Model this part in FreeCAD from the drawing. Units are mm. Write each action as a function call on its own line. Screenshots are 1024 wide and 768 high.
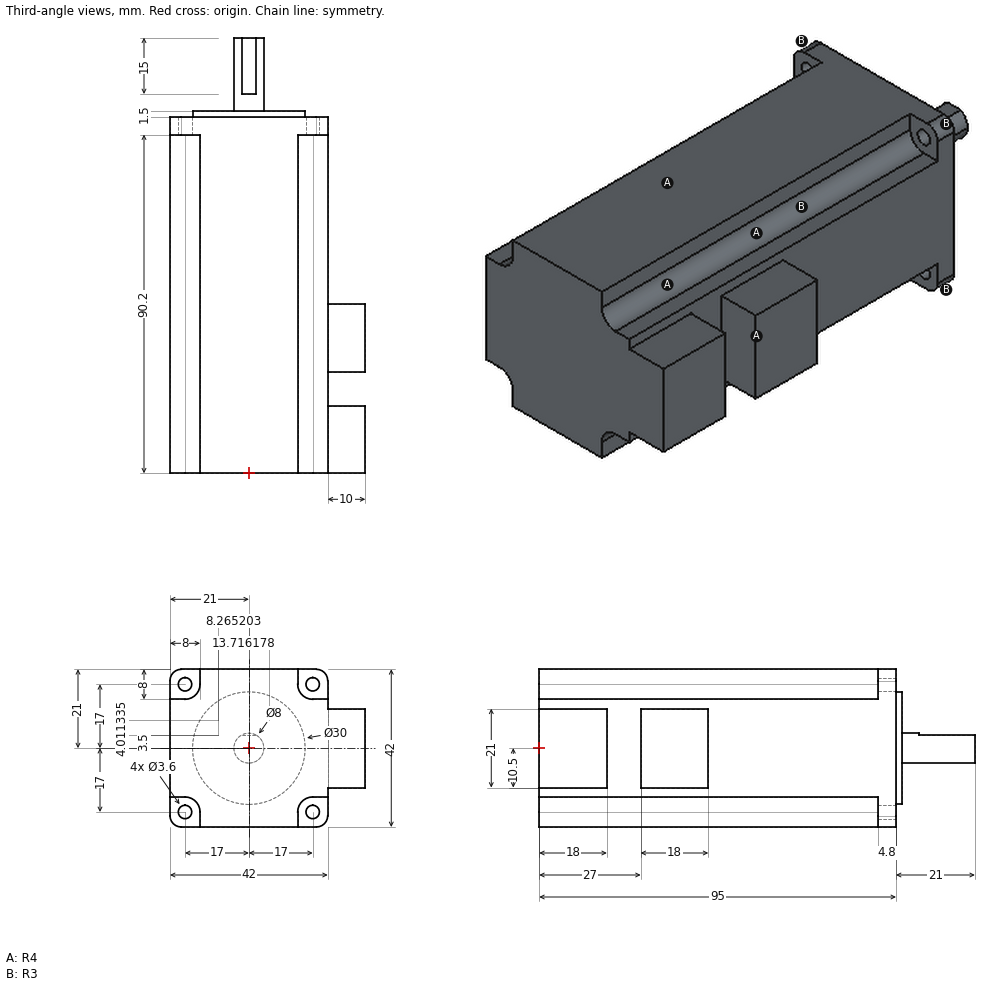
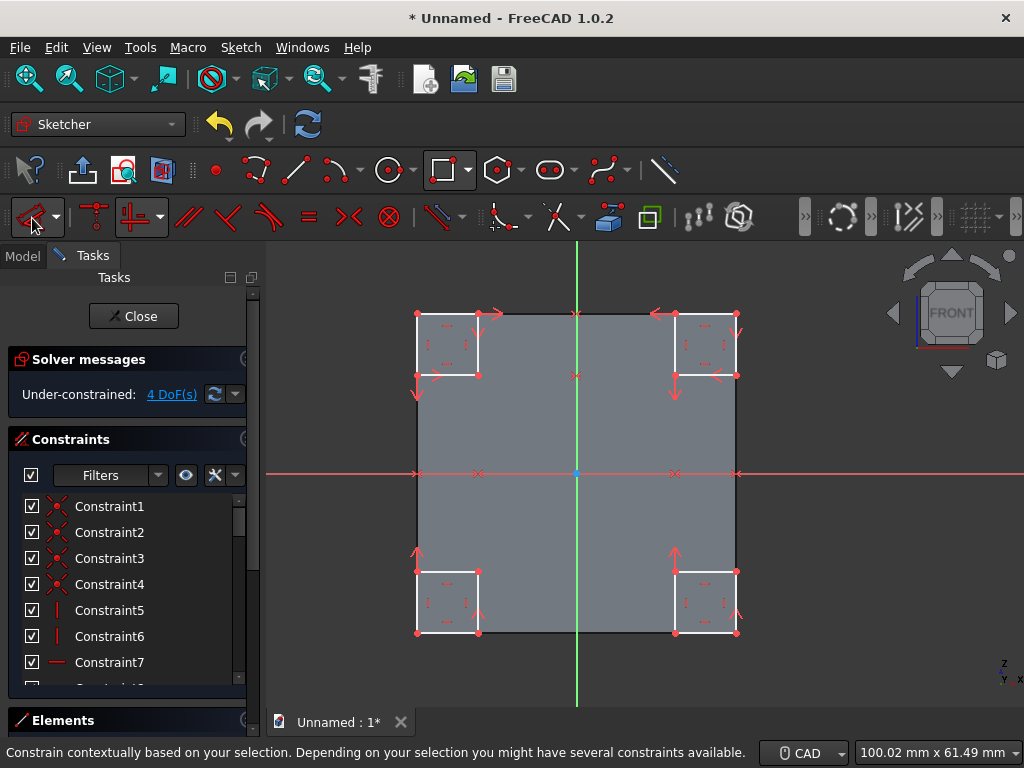
click(417, 332)
click(383, 345)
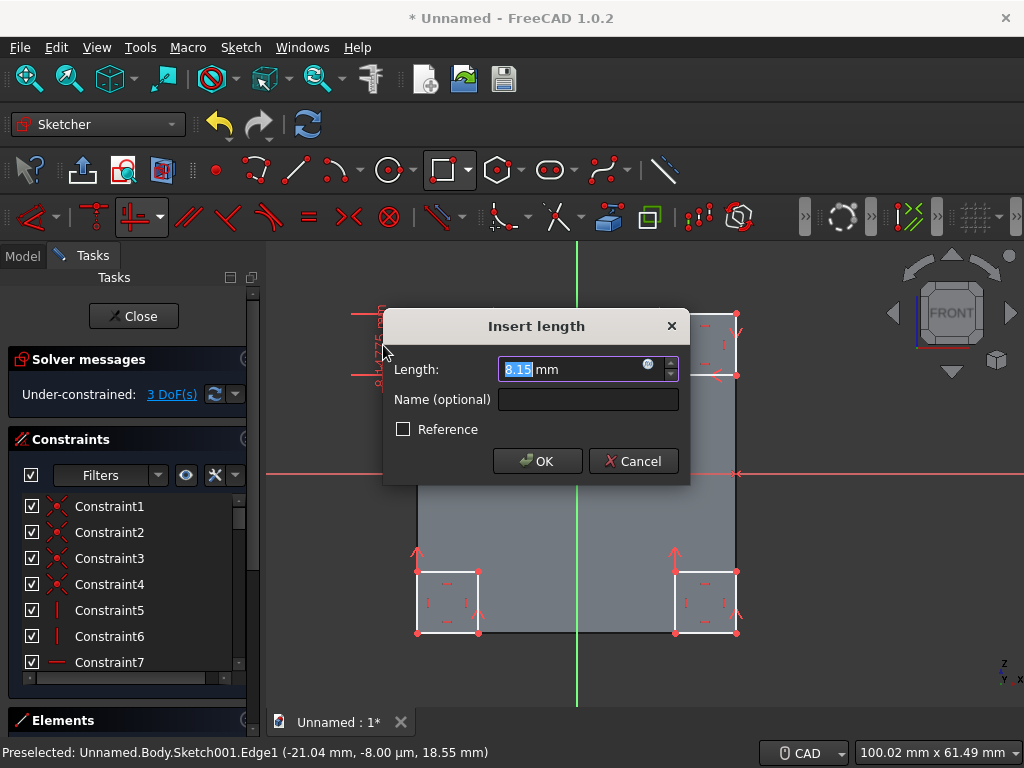
text(8)
key(Return)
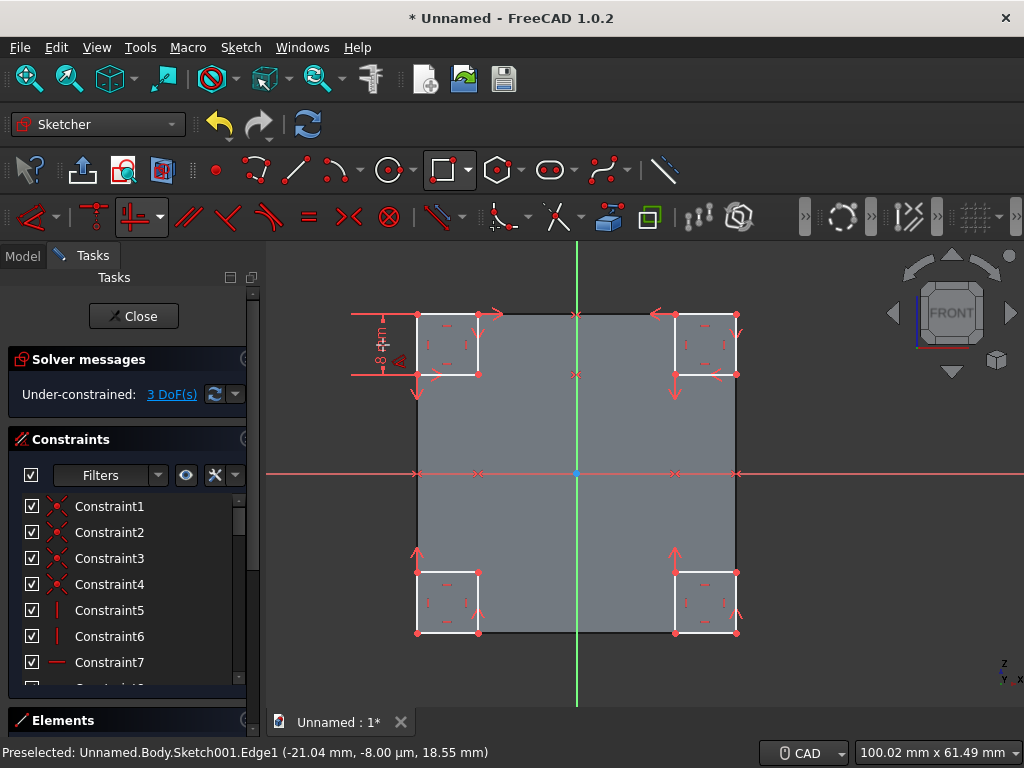
click(435, 375)
click(462, 341)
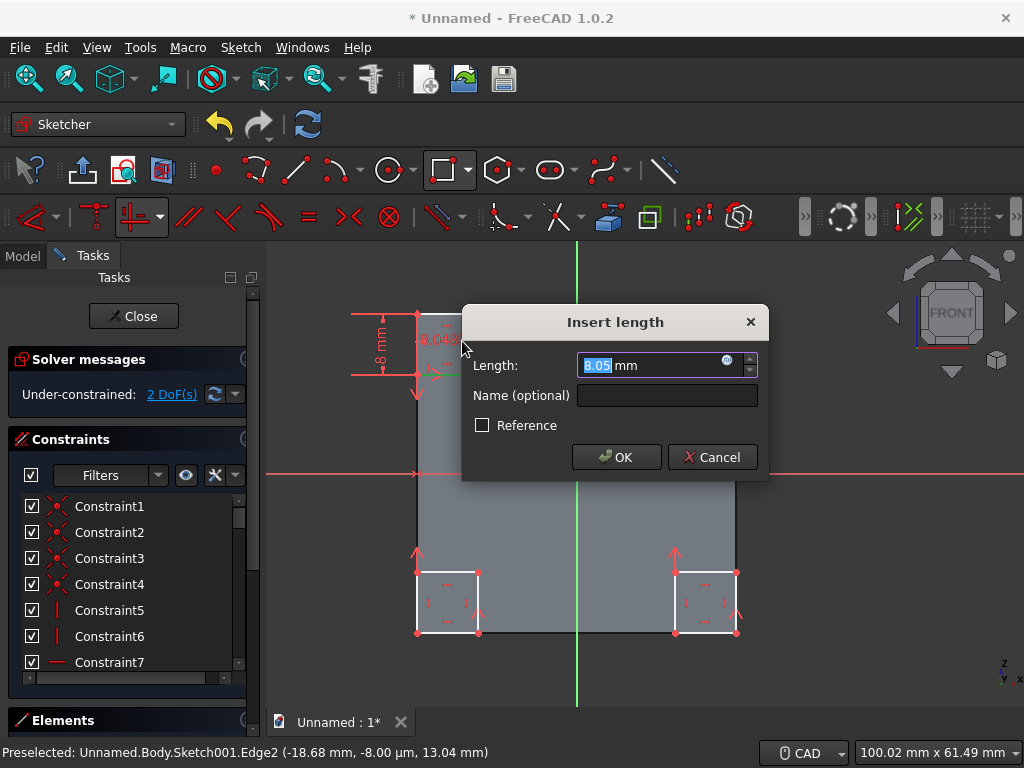
text(8)
key(Return)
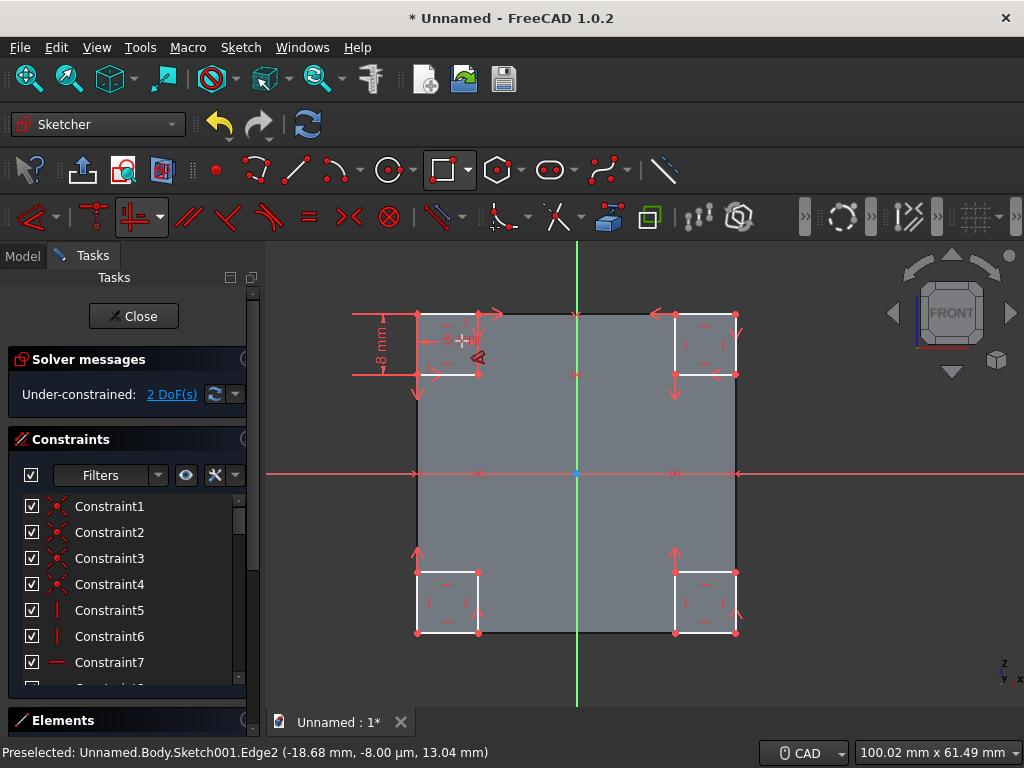
click(417, 314)
click(497, 280)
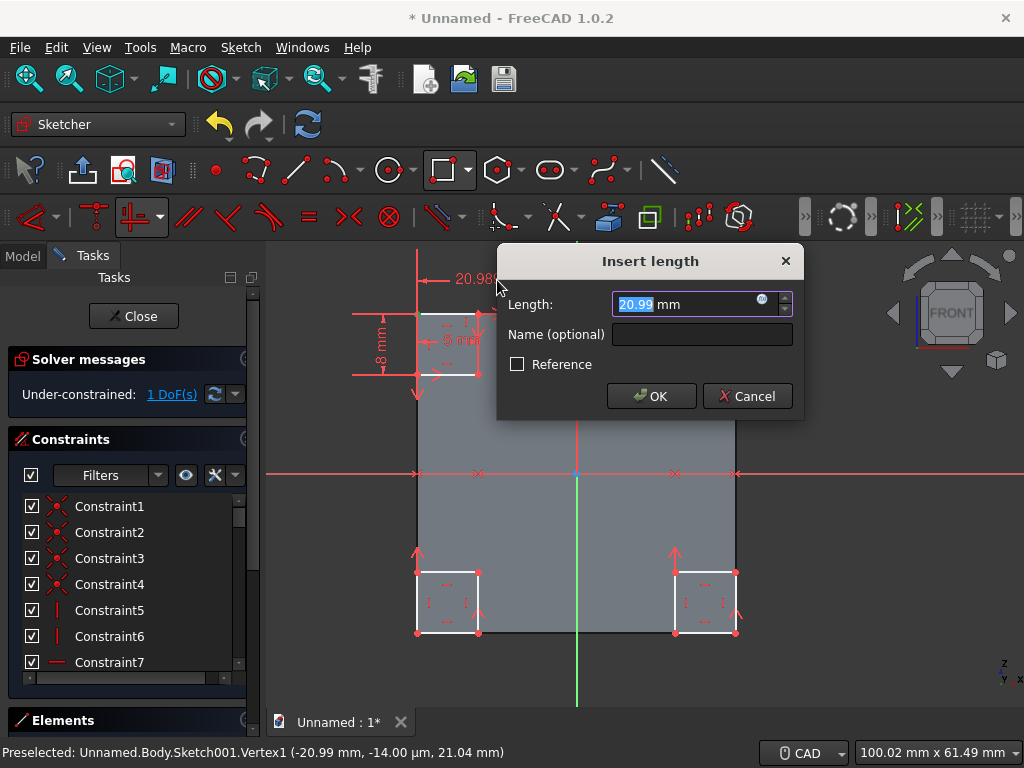
text(21)
key(Return)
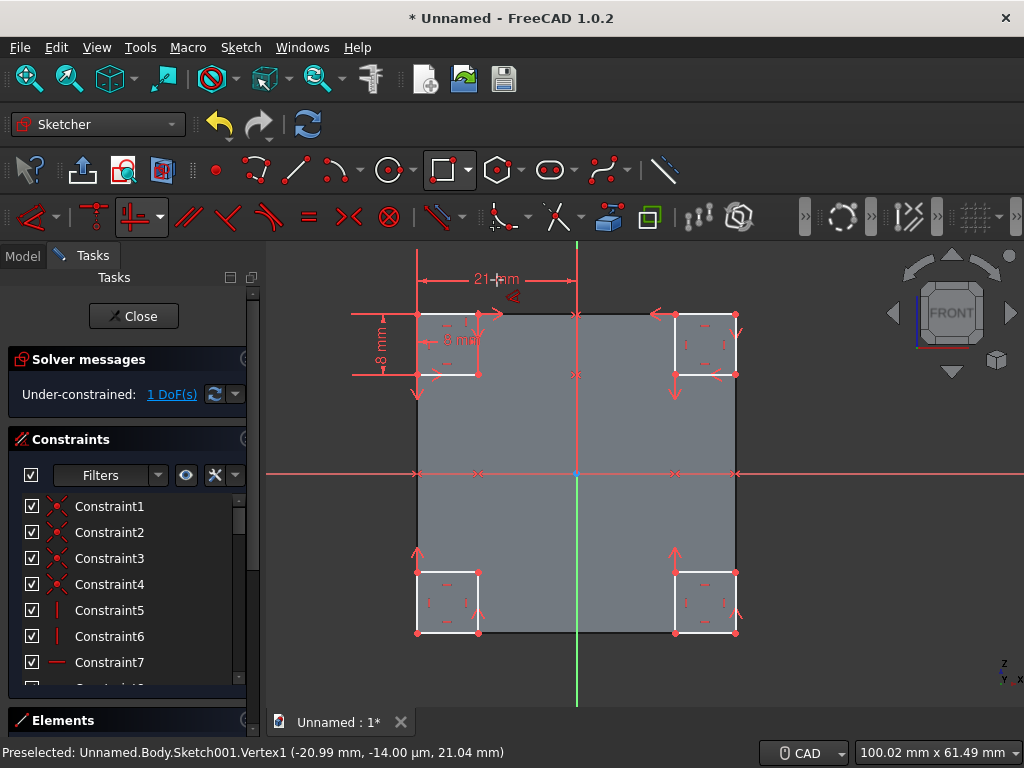
click(417, 314)
click(383, 394)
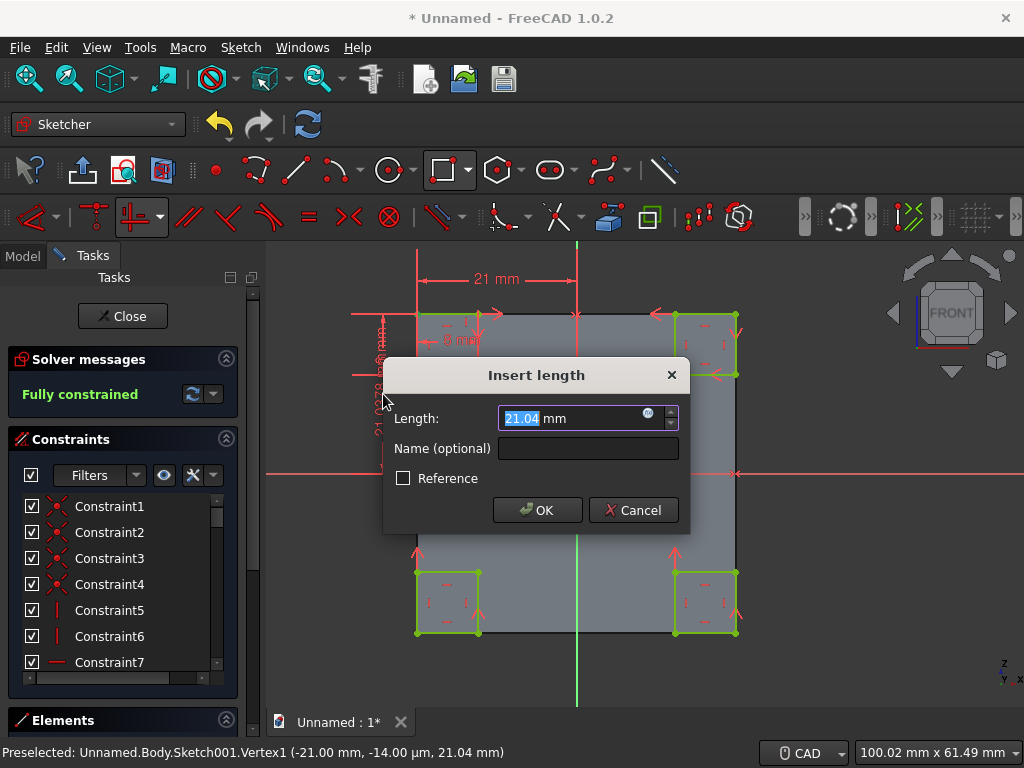
text(21)
key(Return)
key(Escape)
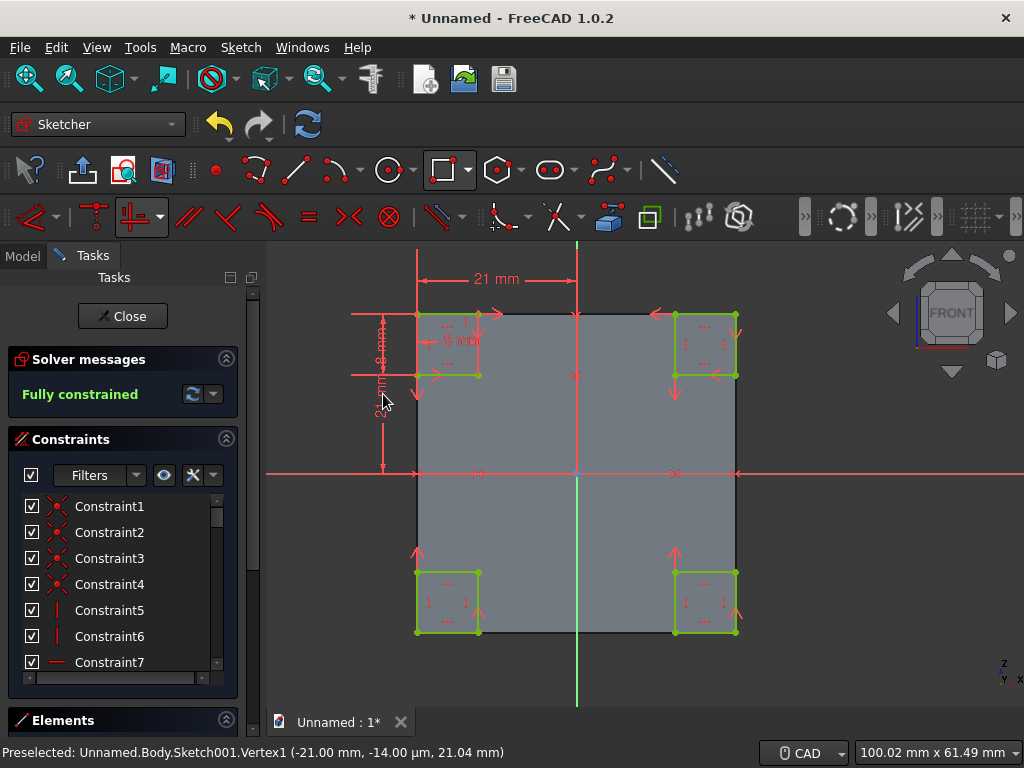
click(123, 316)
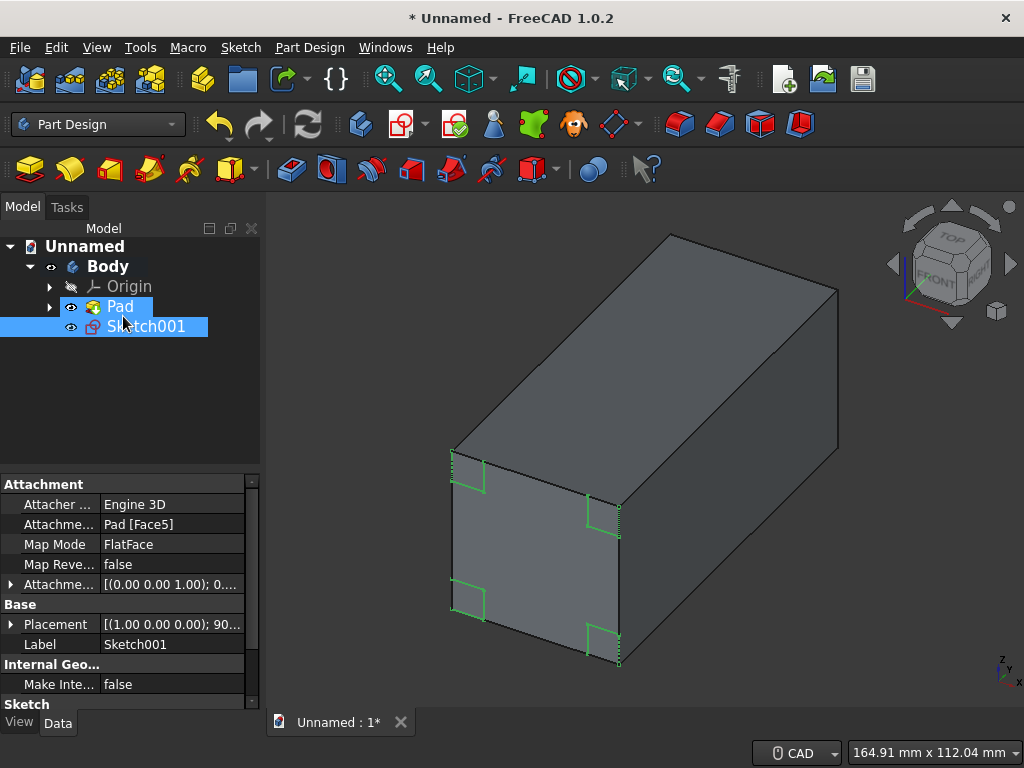
click(292, 170)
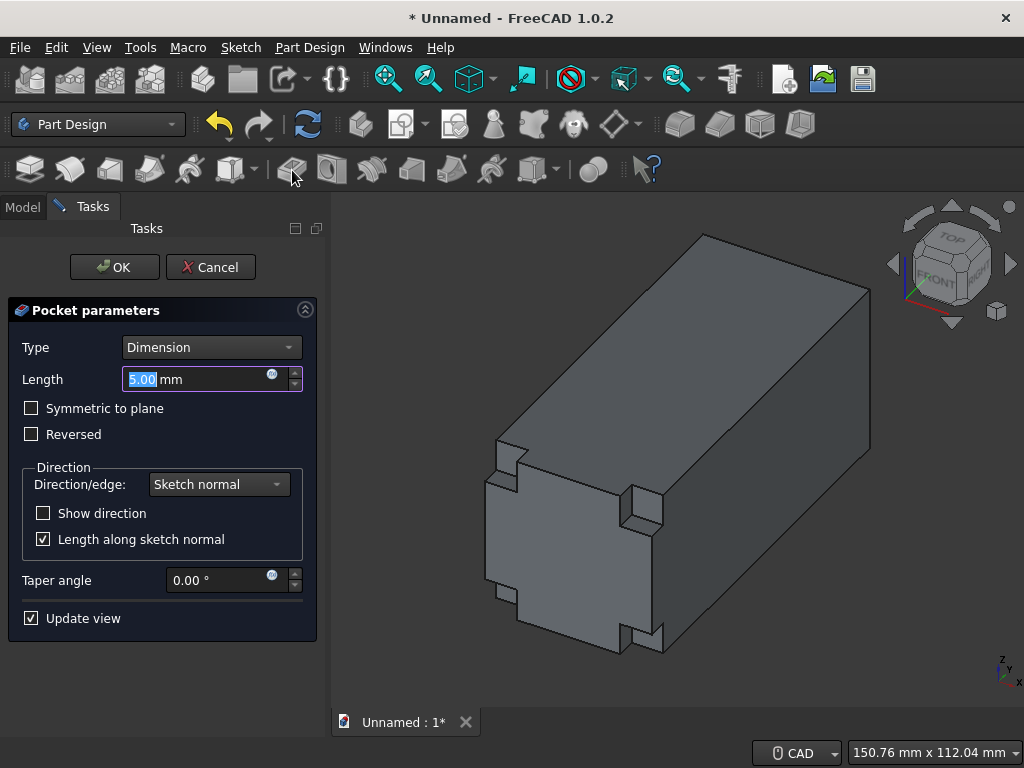
text(90.2)
key(Tab)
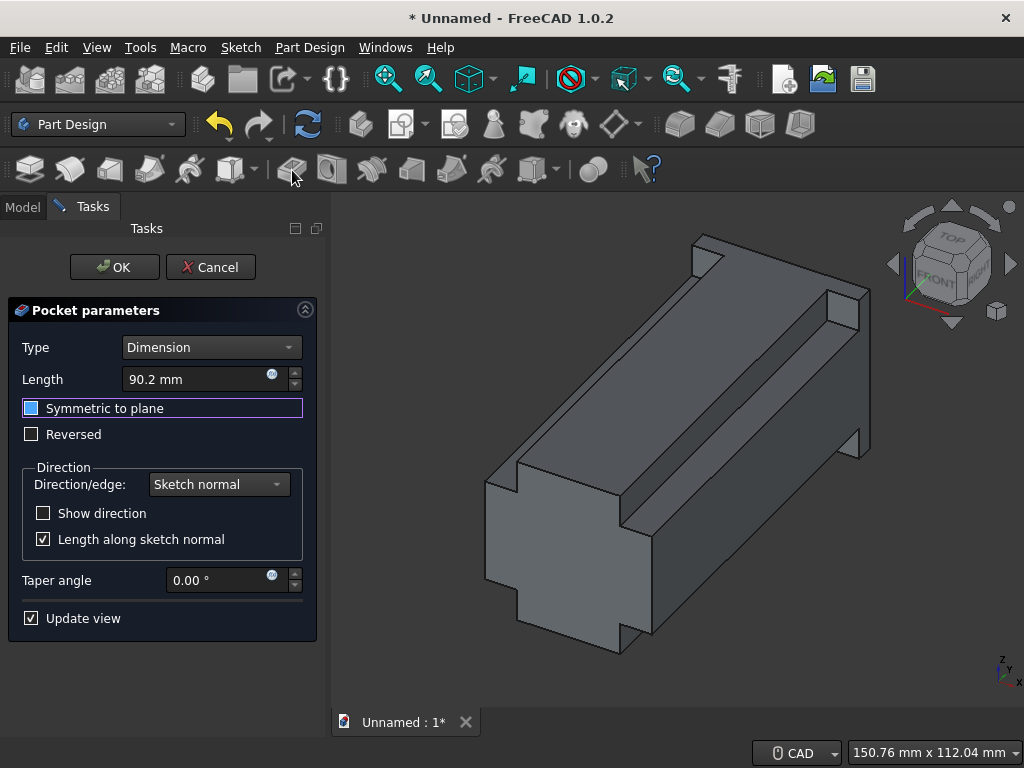
click(115, 267)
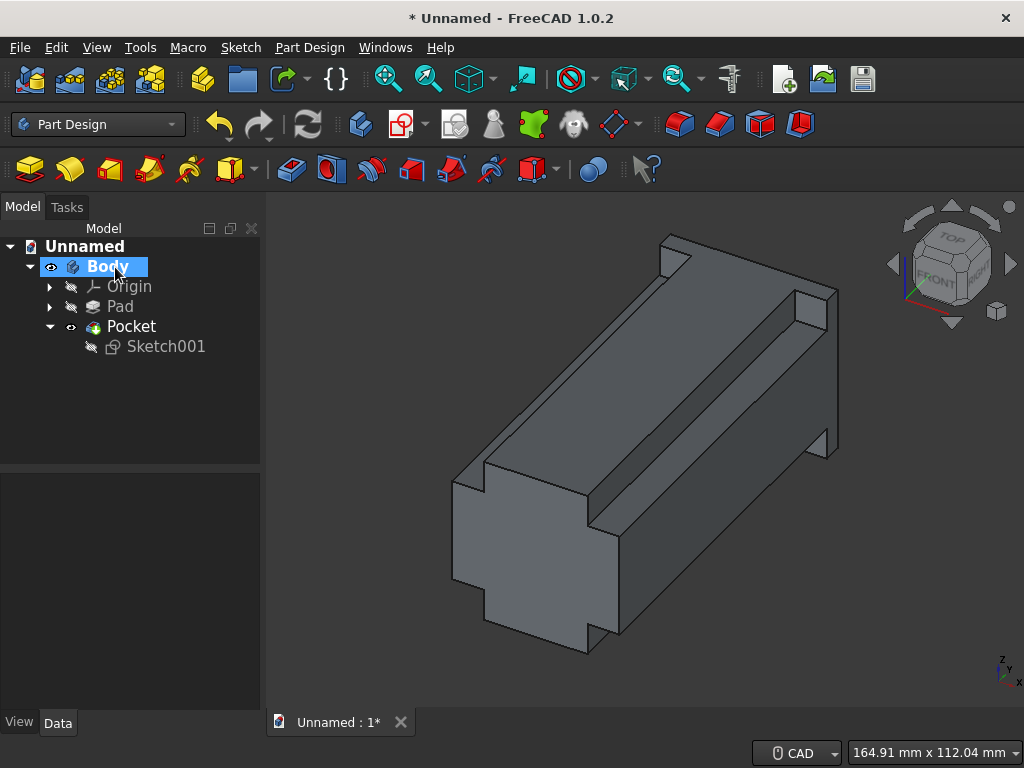
key(4)